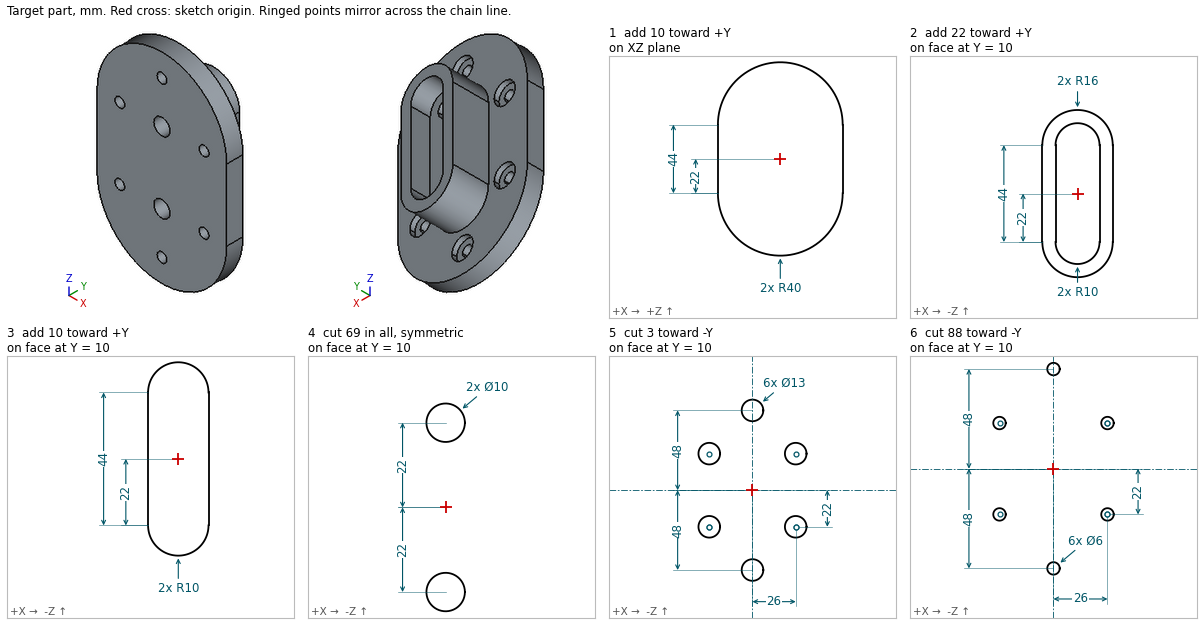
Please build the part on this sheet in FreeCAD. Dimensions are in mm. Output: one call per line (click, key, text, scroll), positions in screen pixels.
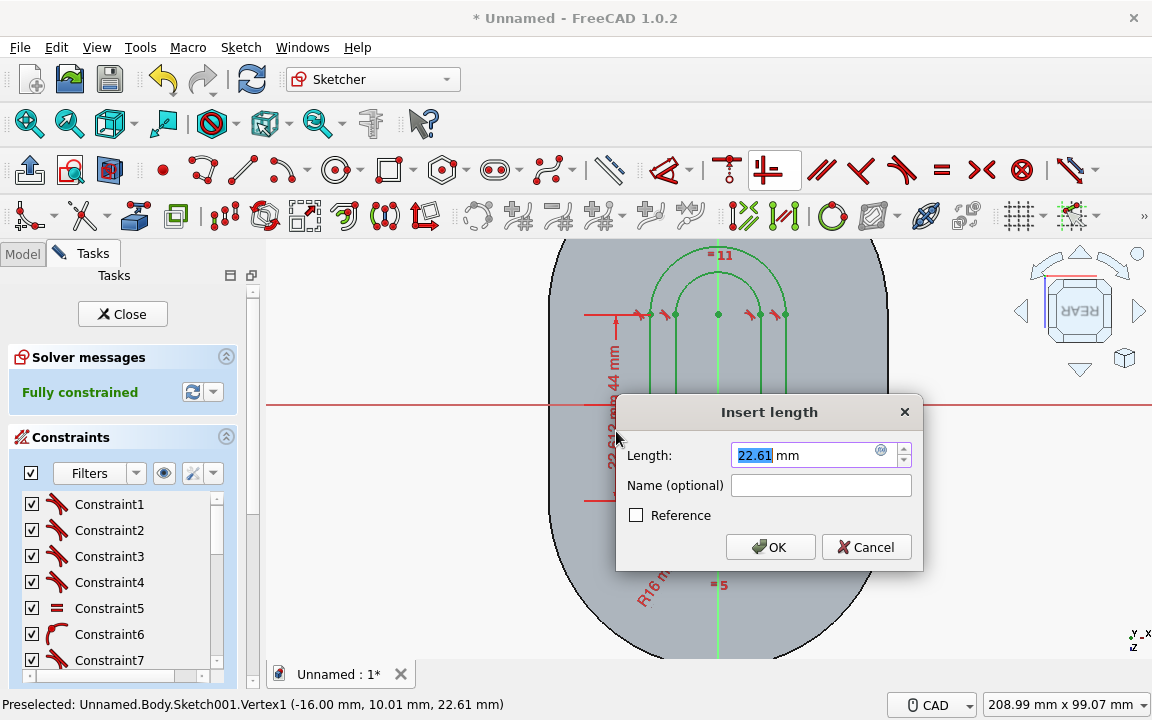
text(22)
key(Return)
key(Escape)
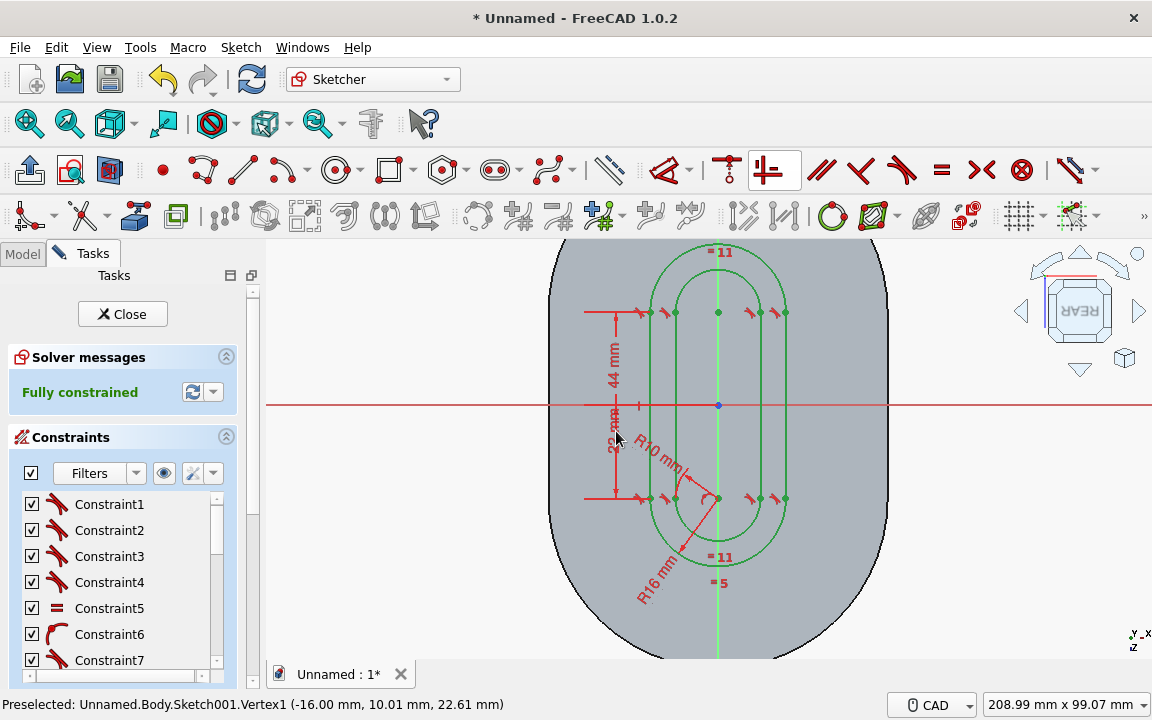
click(123, 314)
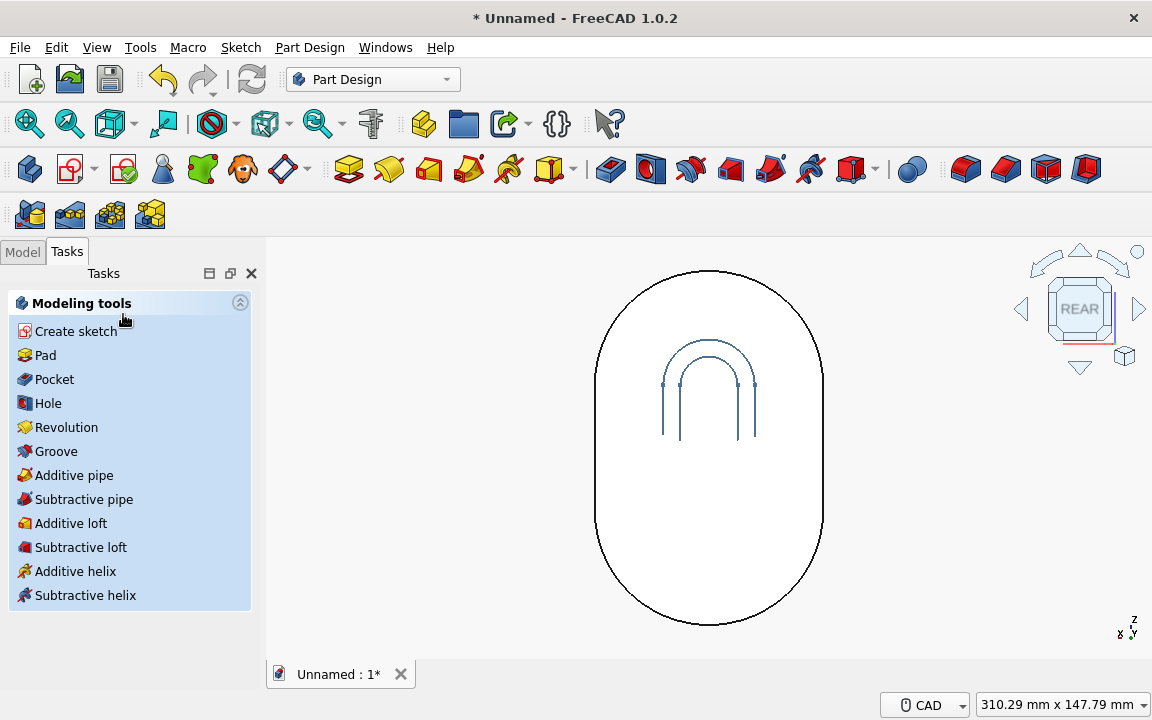
click(350, 170)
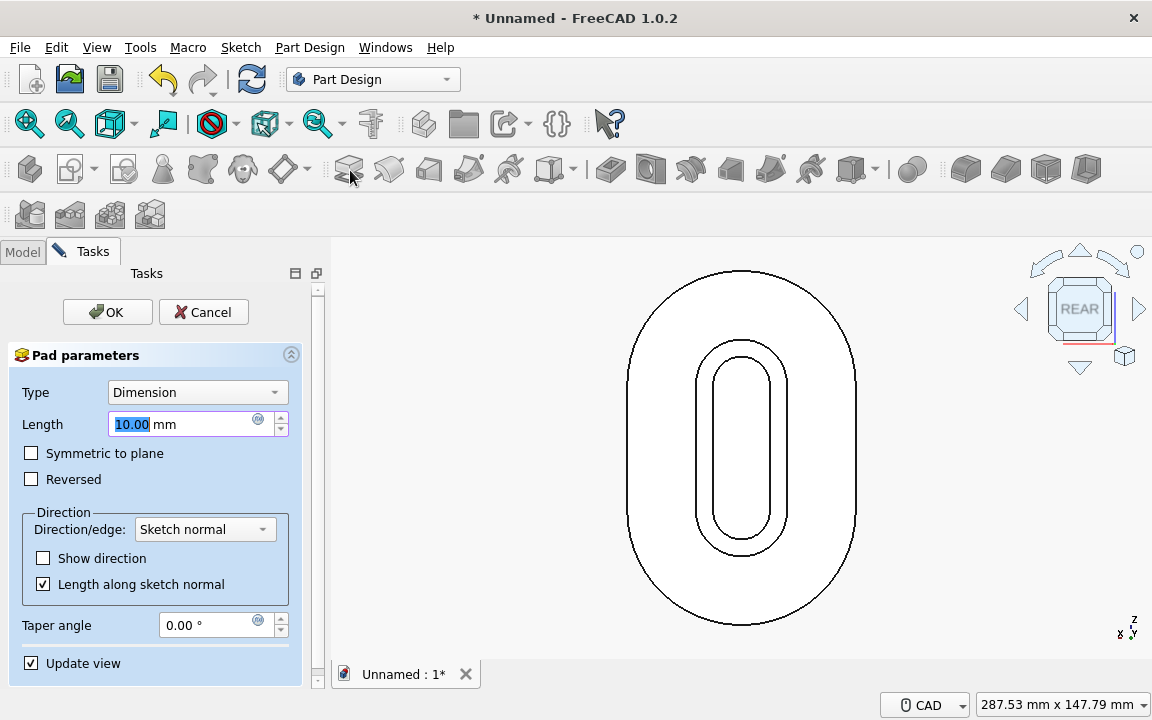
text(22)
key(Tab)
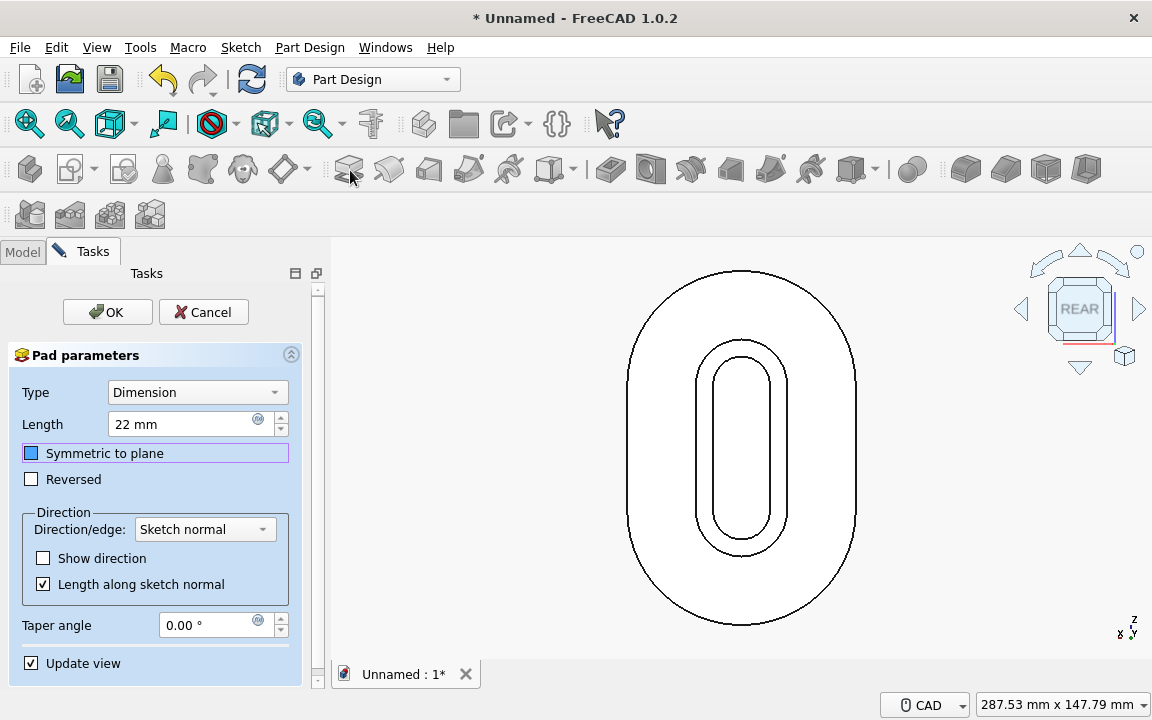
click(108, 312)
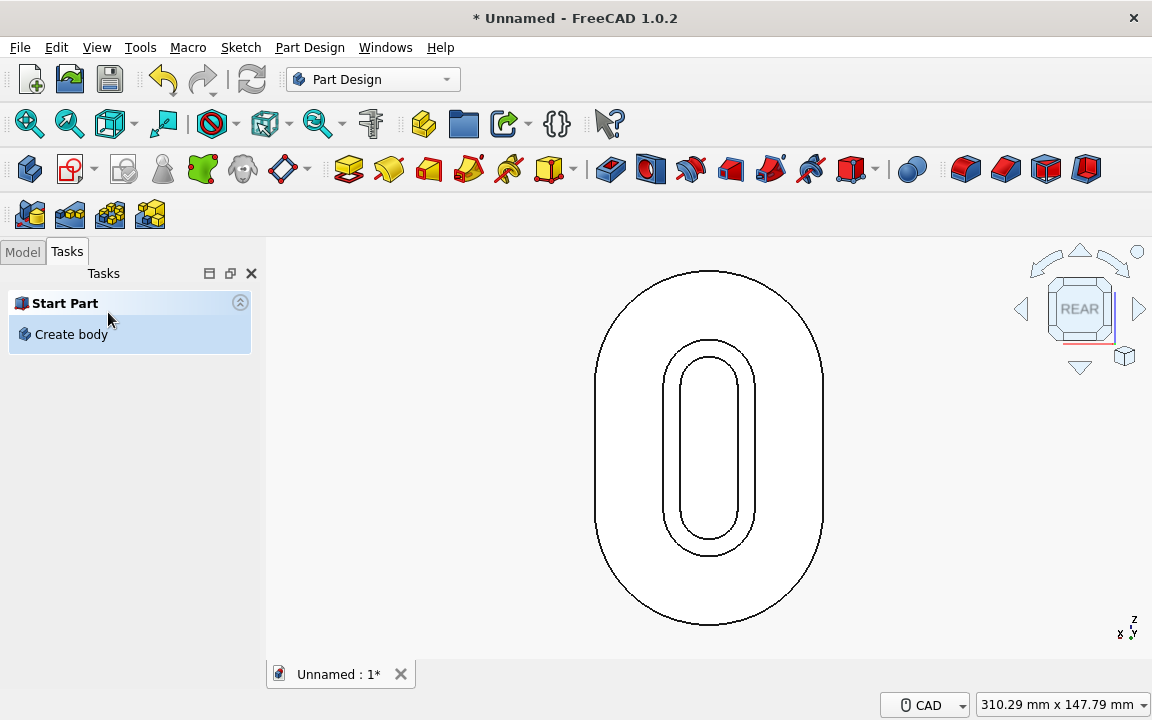
click(644, 548)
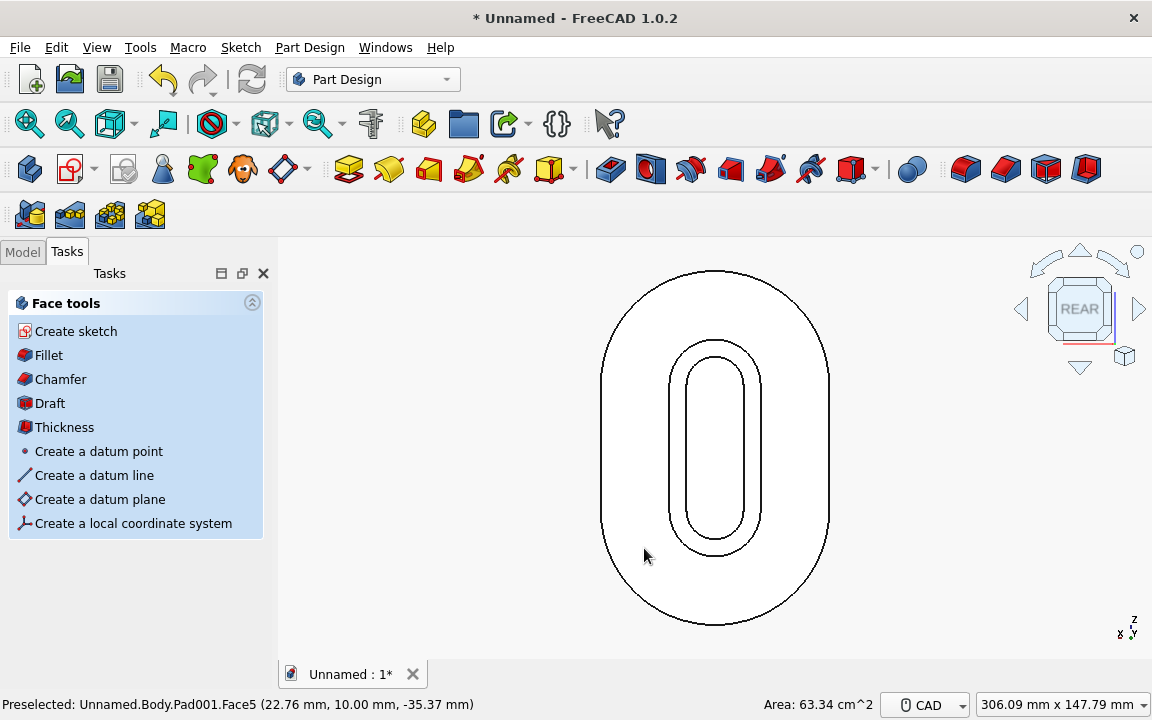
click(70, 170)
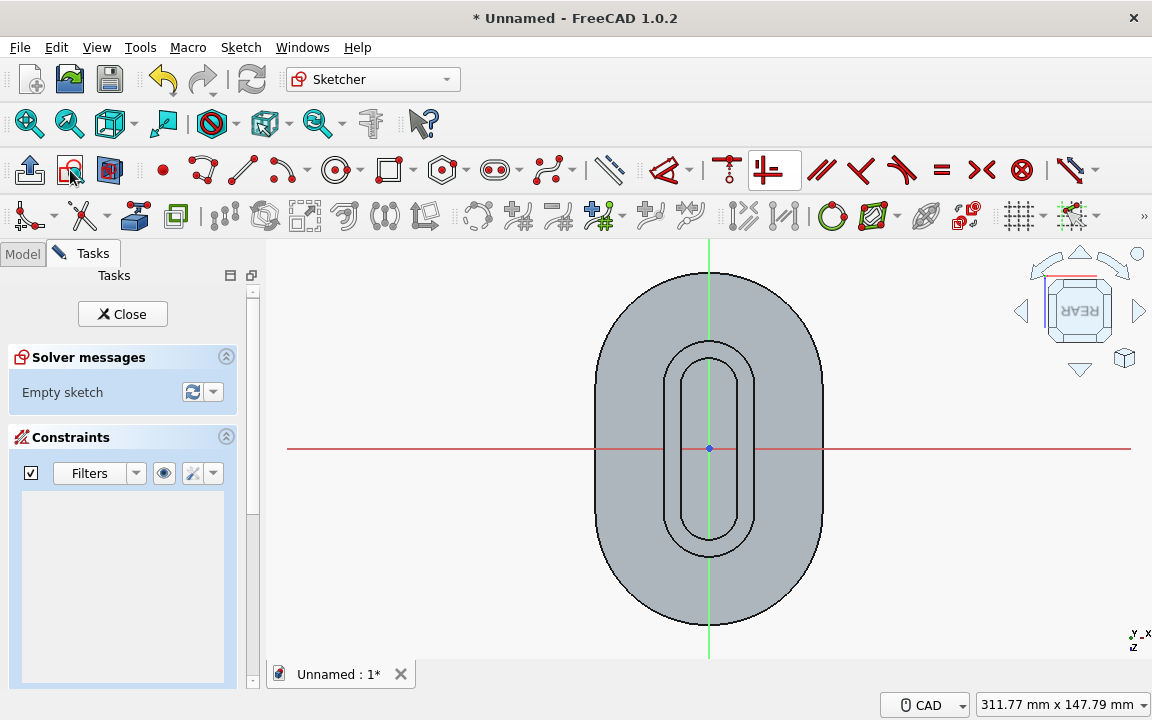
scroll(848, 449, up, 2)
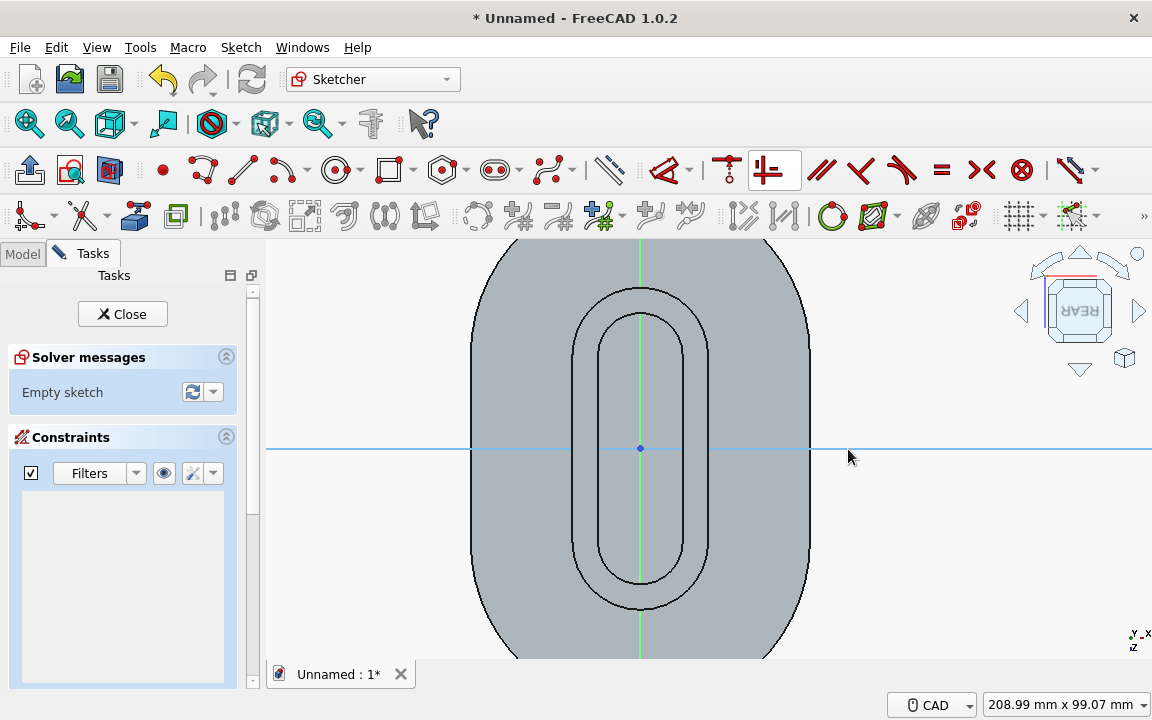
click(496, 170)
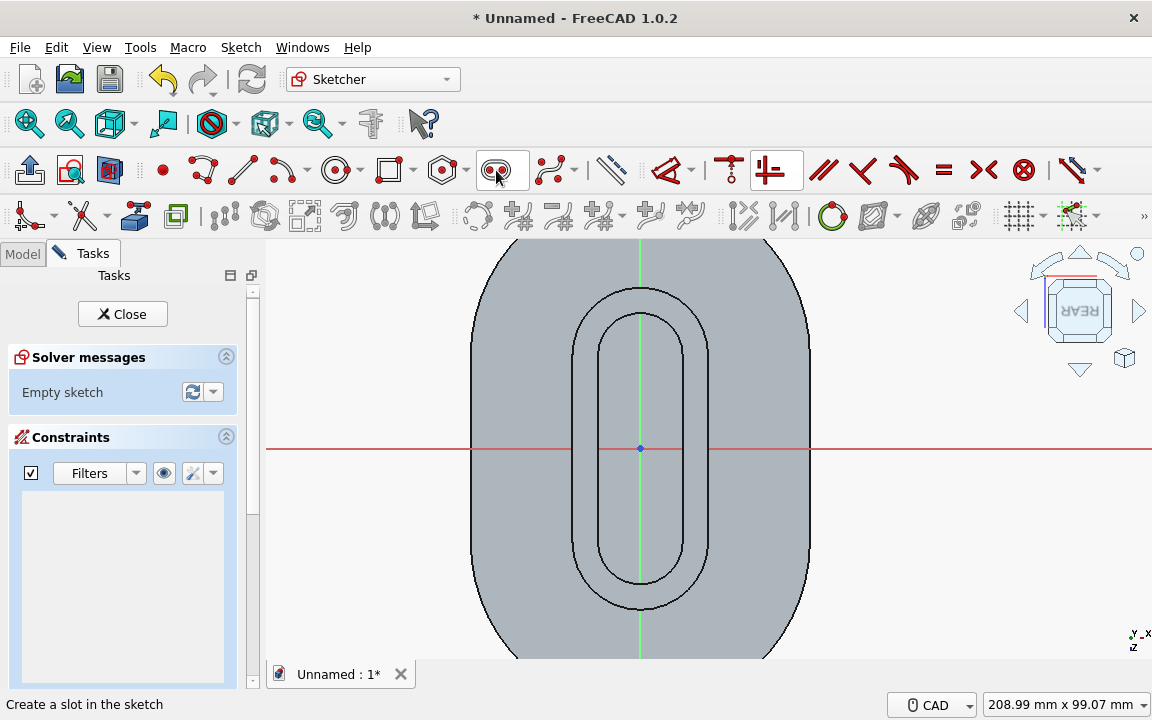
click(640, 542)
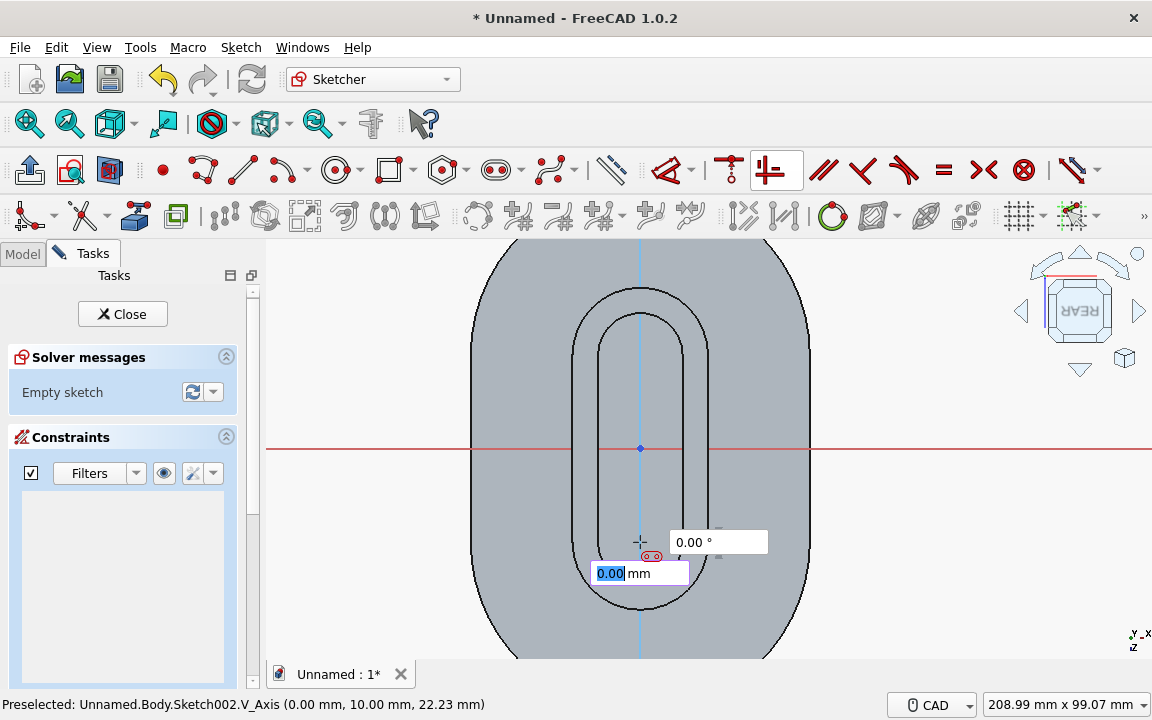
click(649, 355)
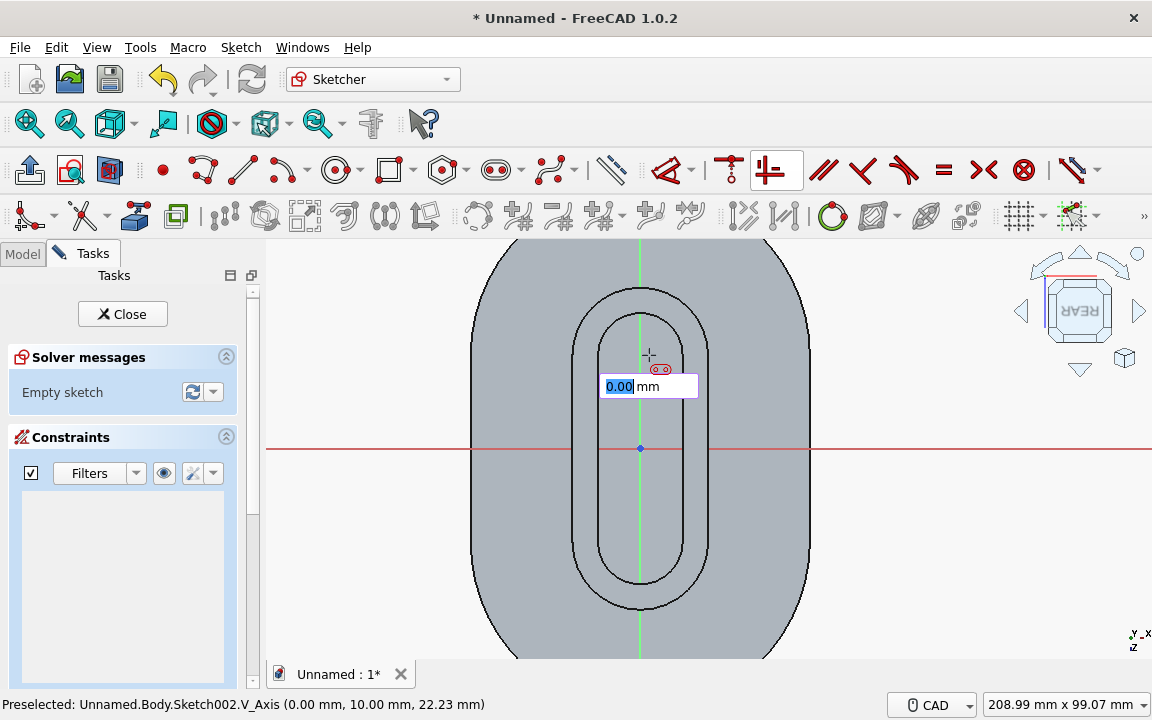
click(598, 421)
key(Escape)